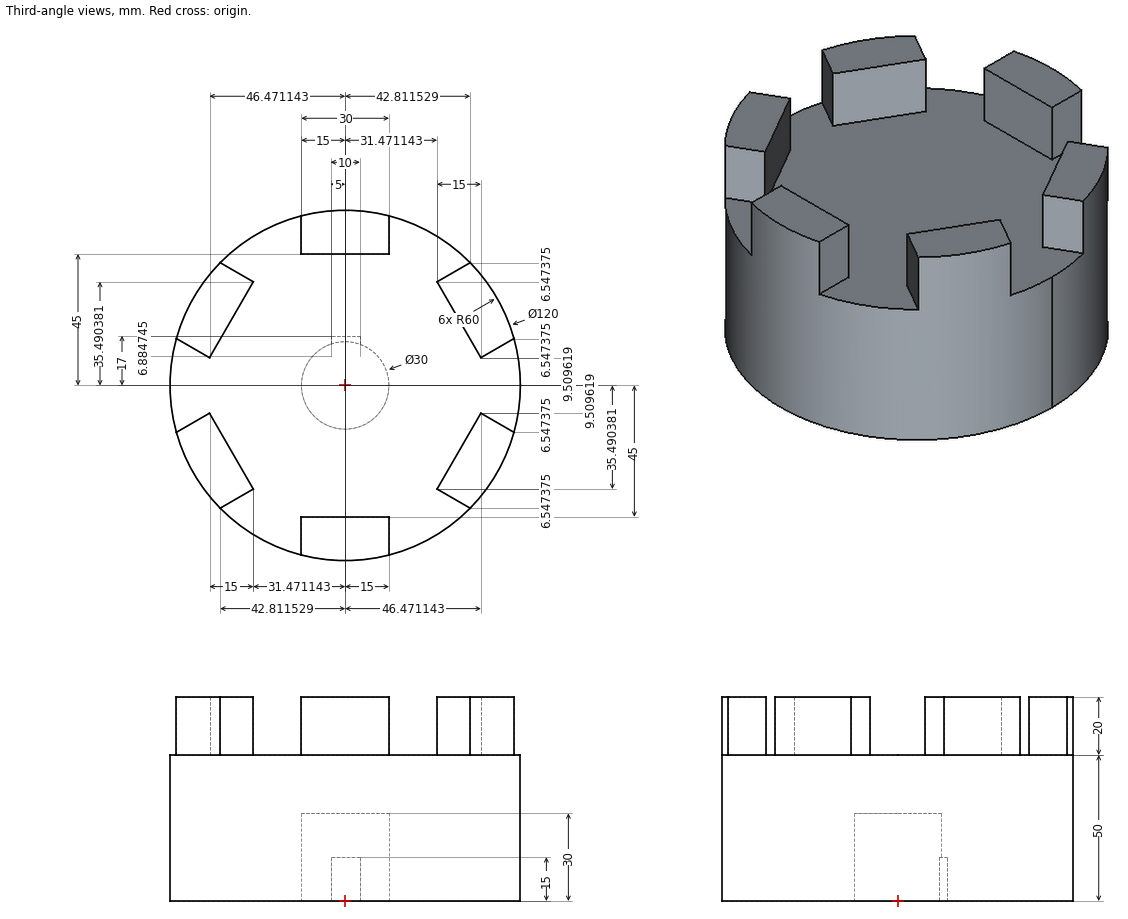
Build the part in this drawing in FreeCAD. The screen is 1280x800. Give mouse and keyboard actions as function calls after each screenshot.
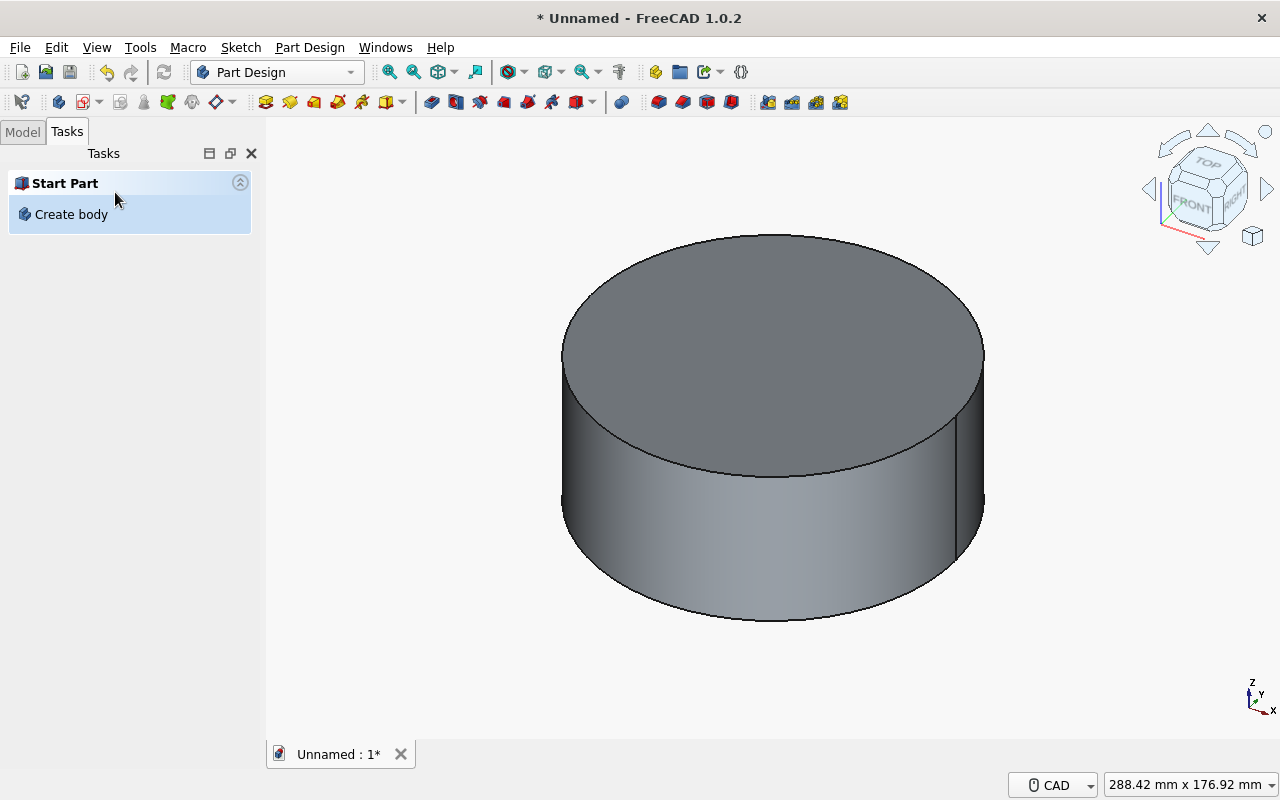
click(773, 355)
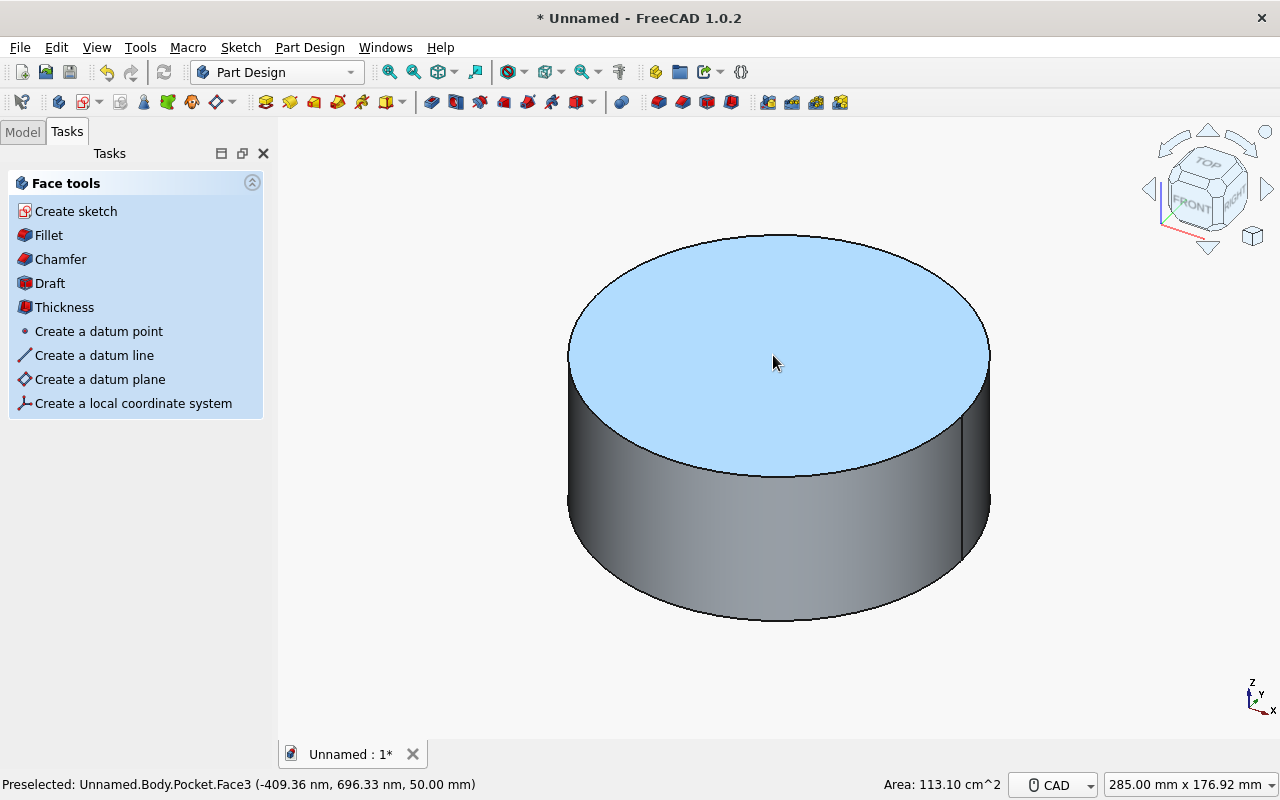
click(84, 102)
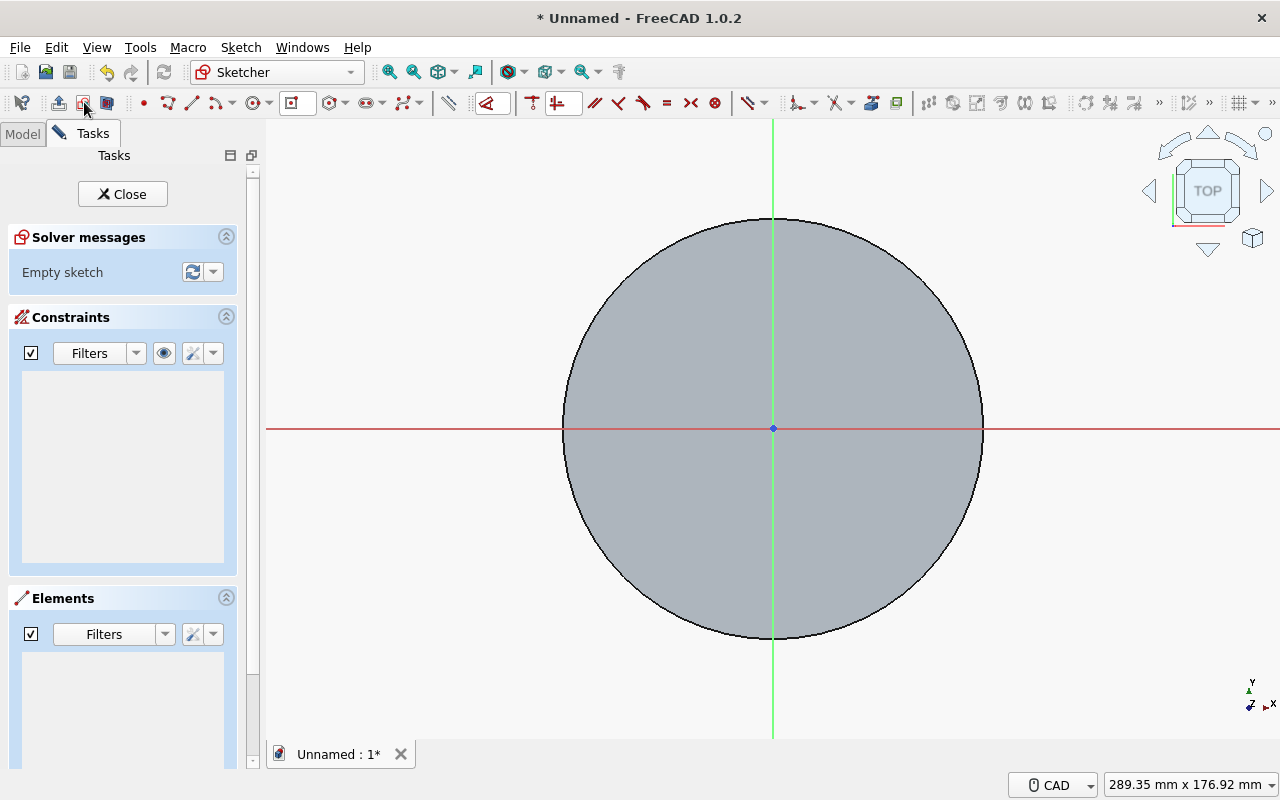
key(g)
key(m)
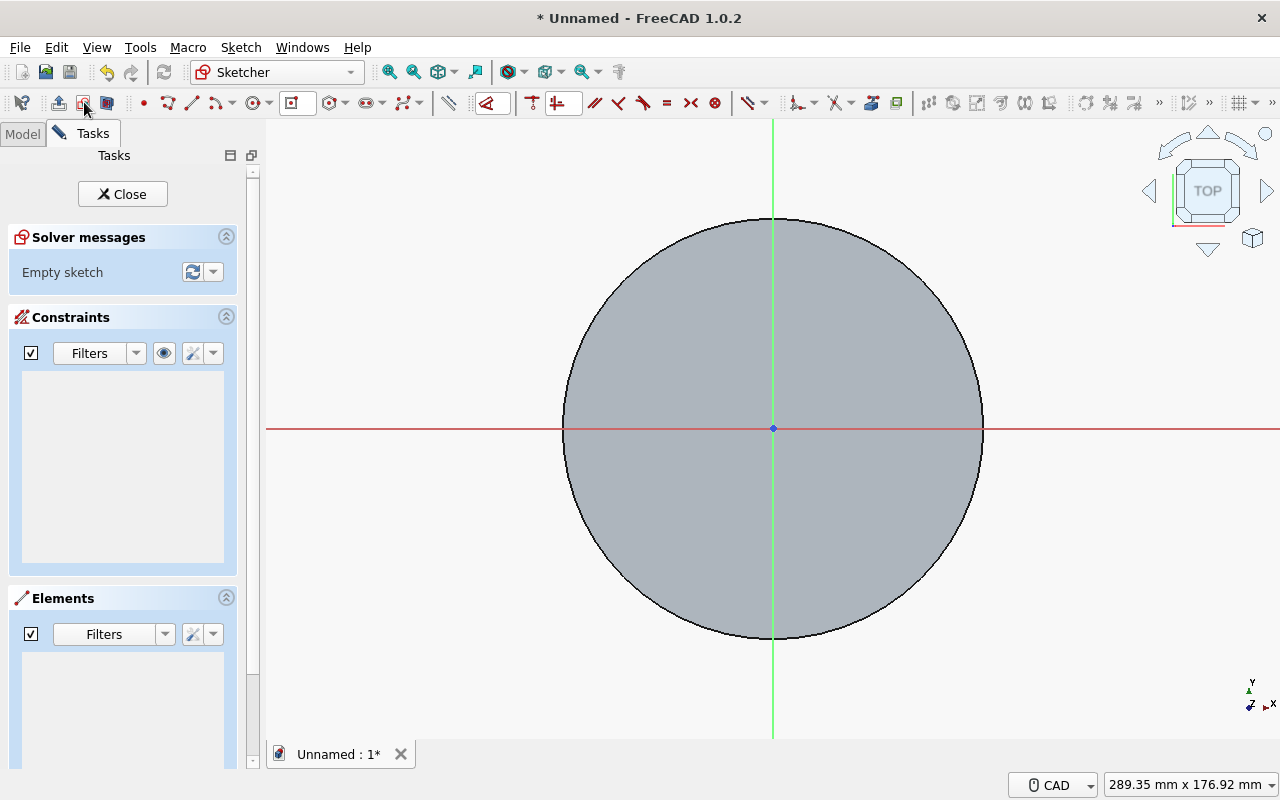
click(923, 282)
click(883, 305)
click(936, 396)
click(976, 373)
right_click(976, 373)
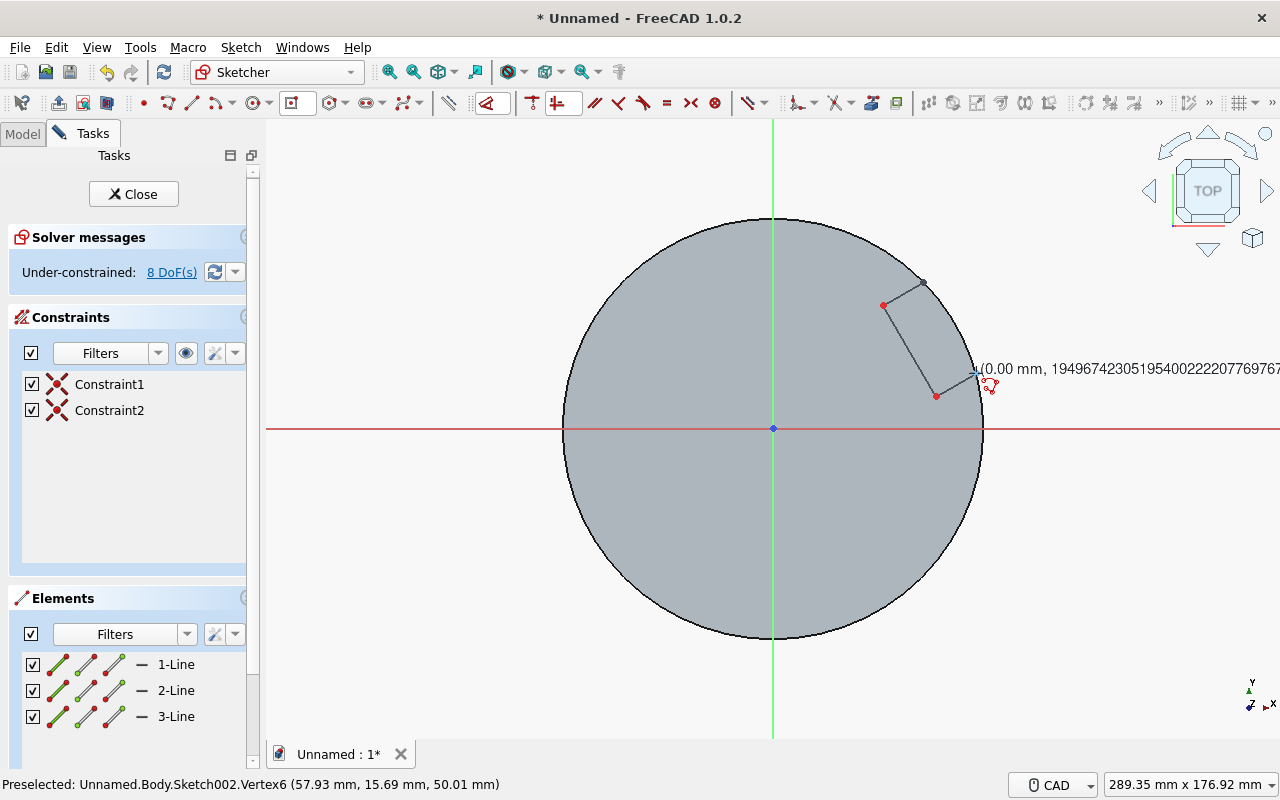
click(234, 104)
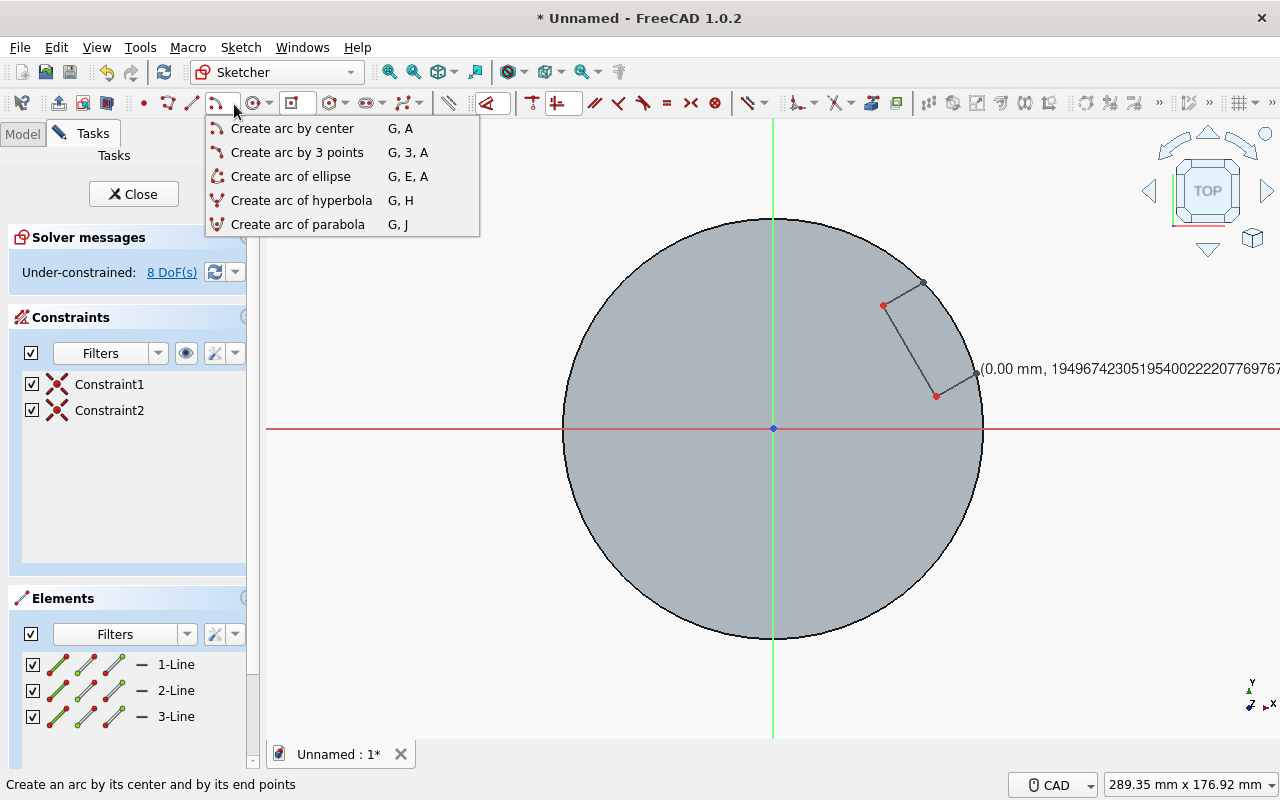
click(342, 152)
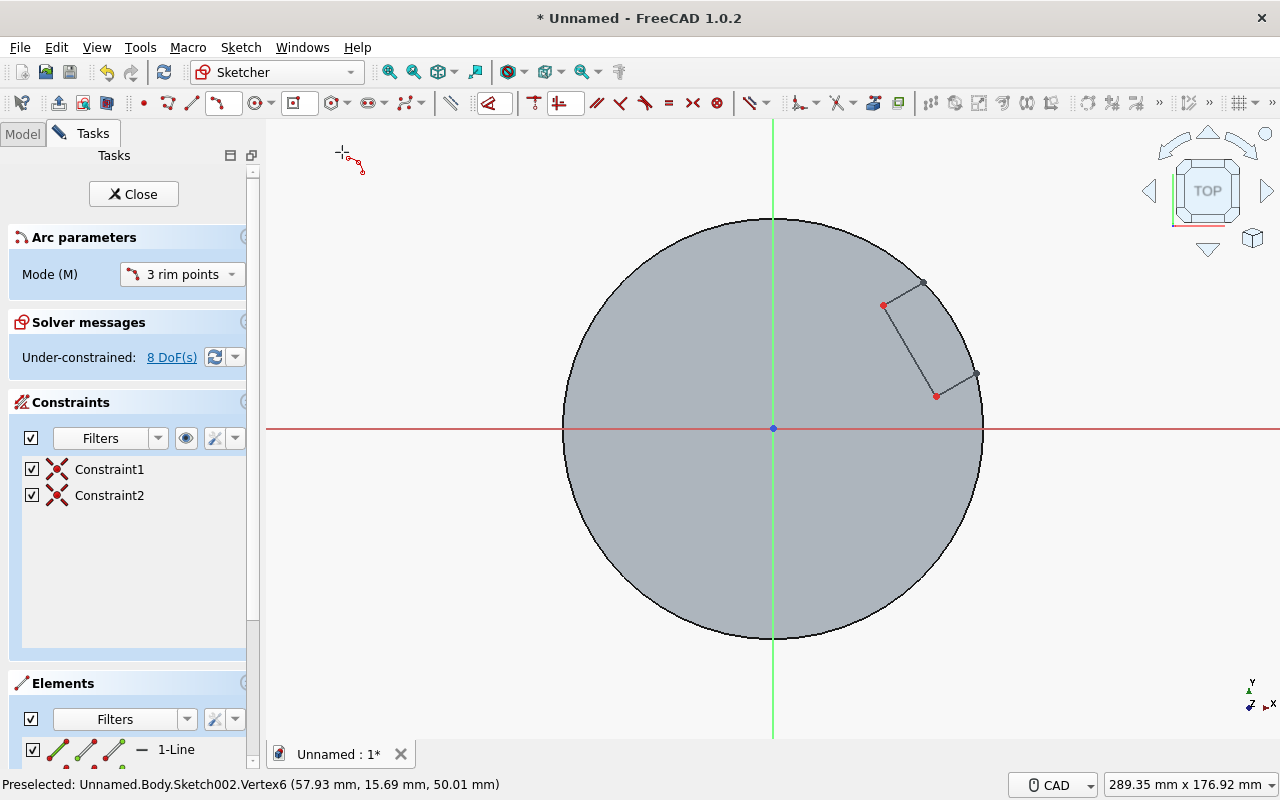
click(976, 374)
click(923, 283)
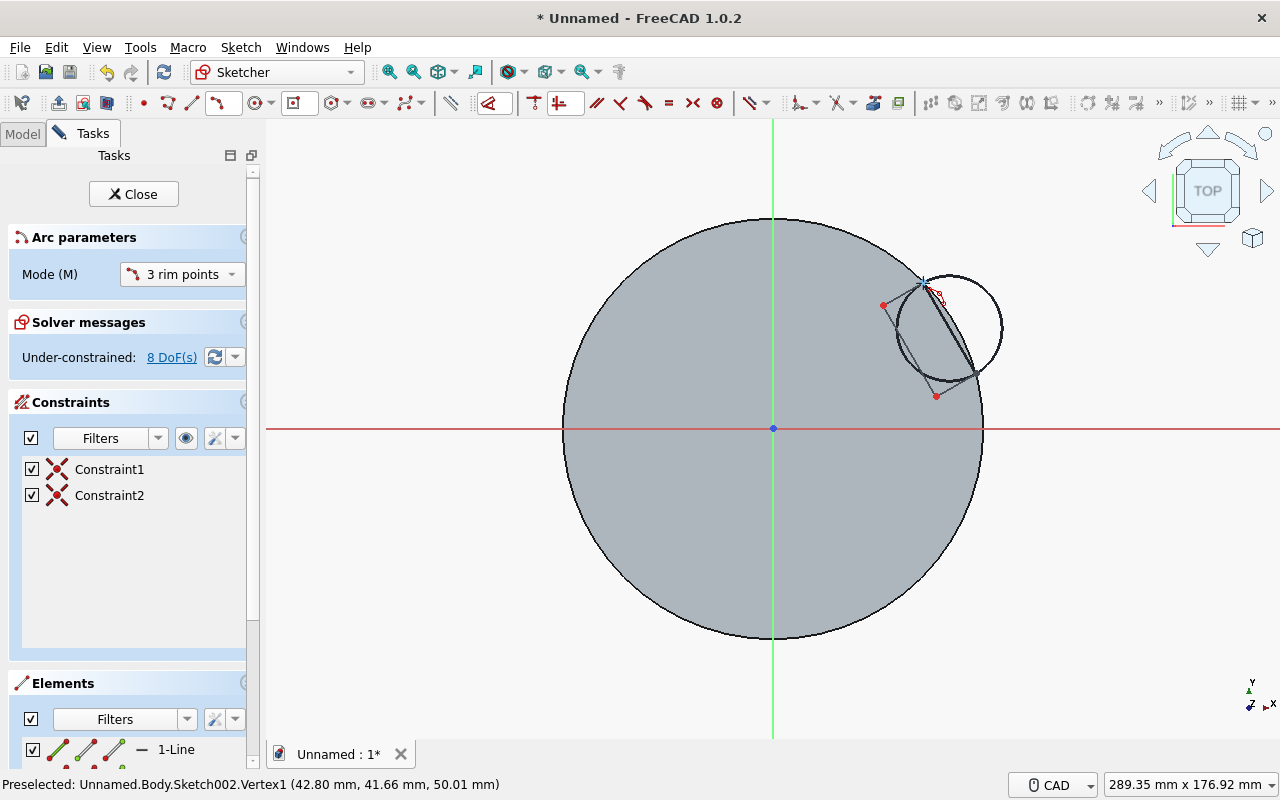
scroll(955, 324, up, 5)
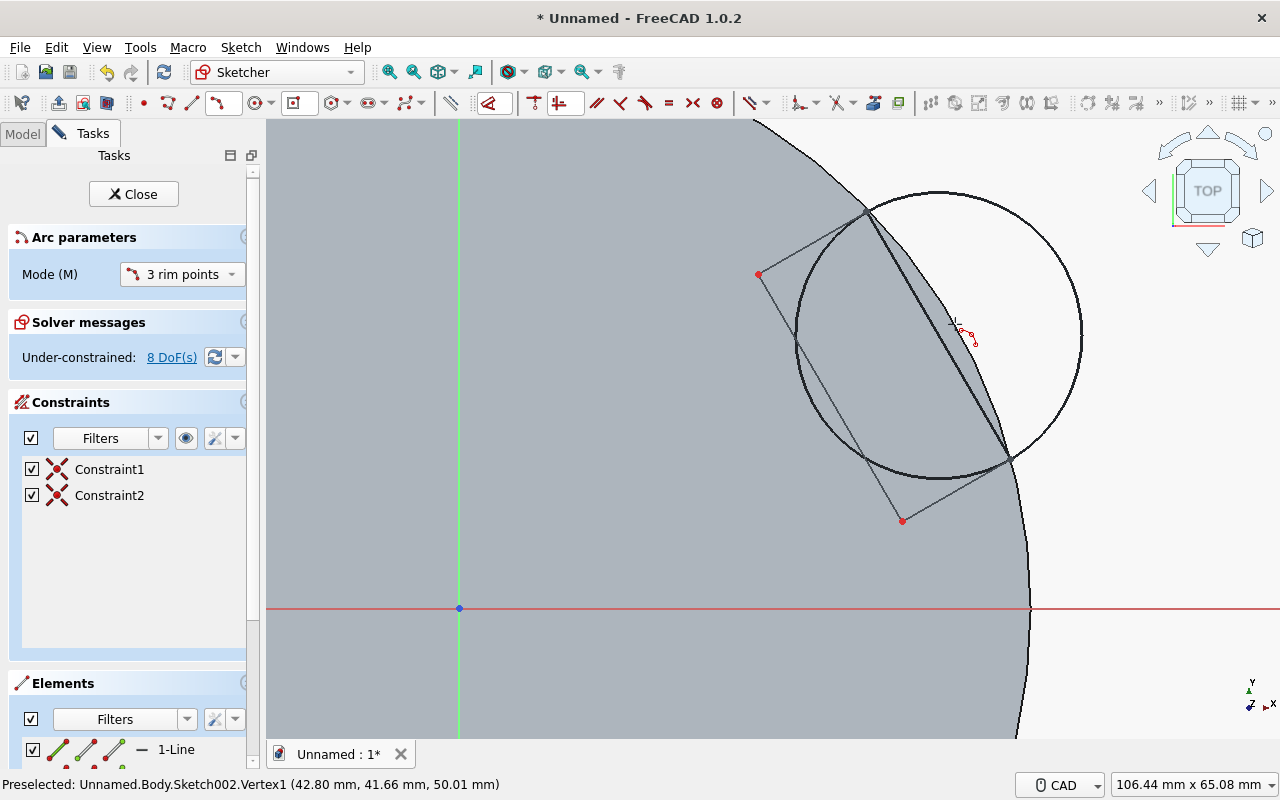
click(954, 323)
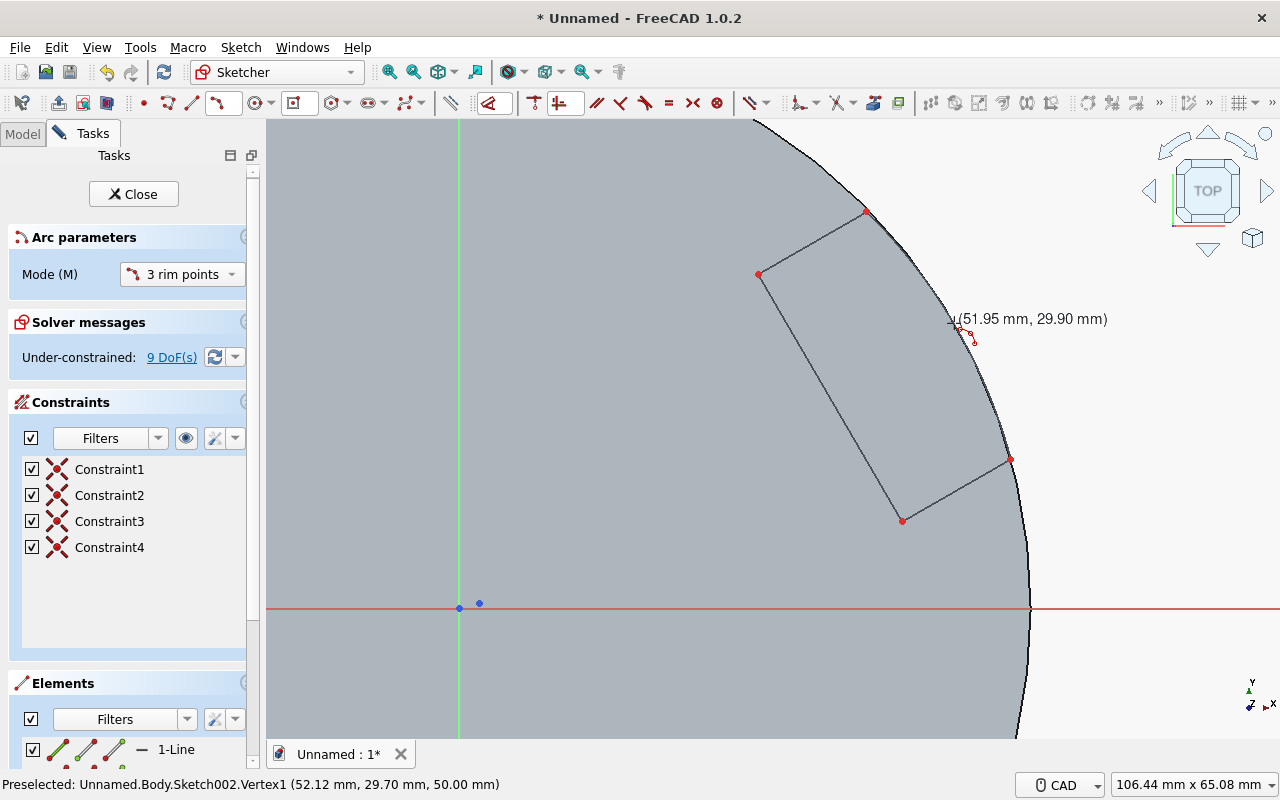
key(g)
key(m)